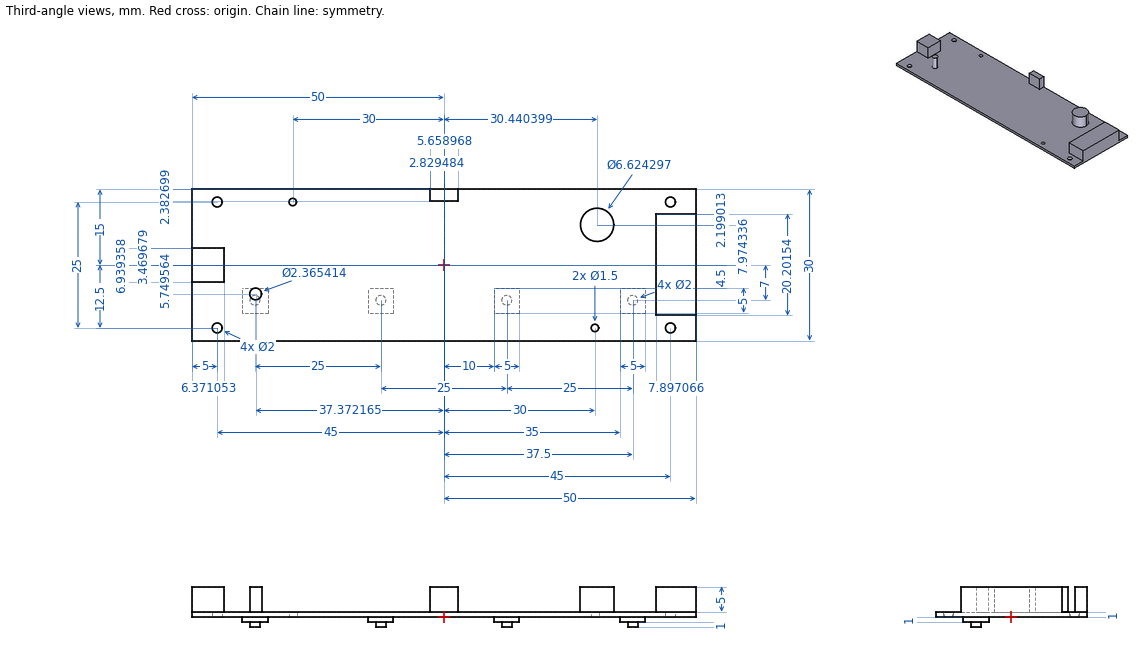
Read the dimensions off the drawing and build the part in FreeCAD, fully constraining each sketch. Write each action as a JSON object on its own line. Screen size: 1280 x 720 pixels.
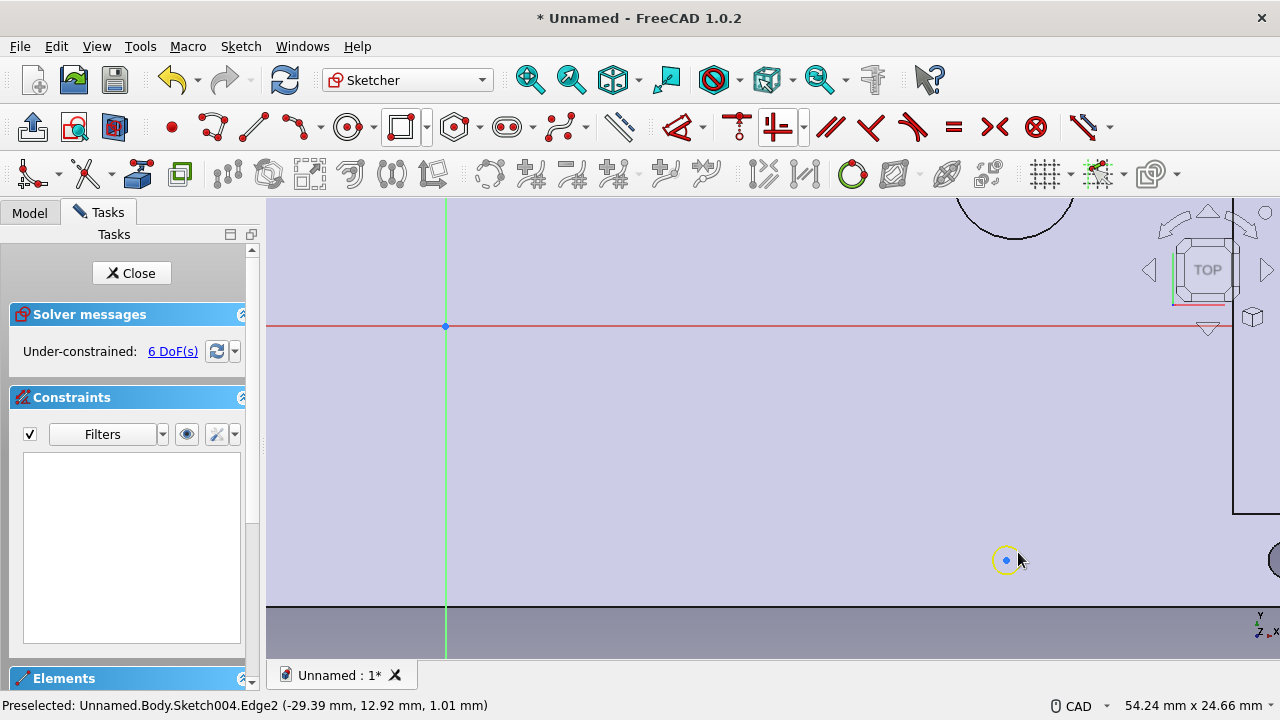
{"action": "left_click", "coordinate": [1017, 550]}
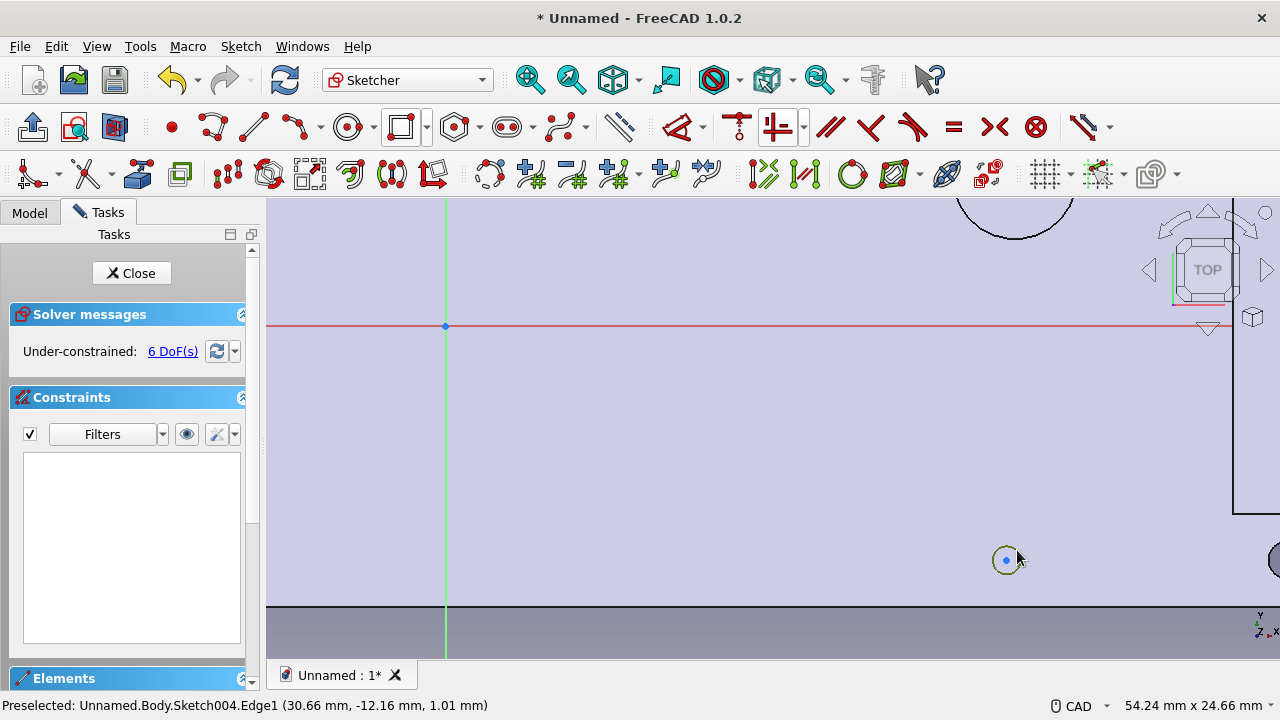
{"action": "scroll", "coordinate": [1019, 553], "scroll_direction": "down", "scroll_amount": 3}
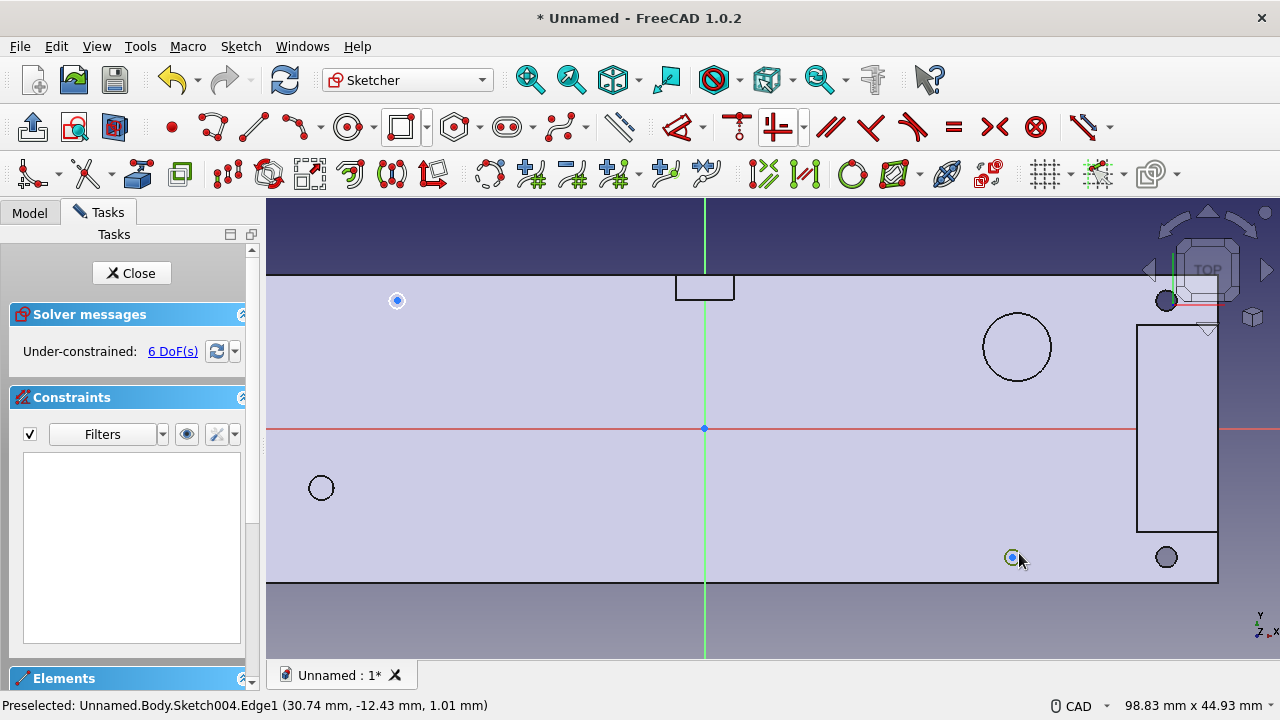
{"action": "scroll", "coordinate": [403, 295], "scroll_direction": "up", "scroll_amount": 3}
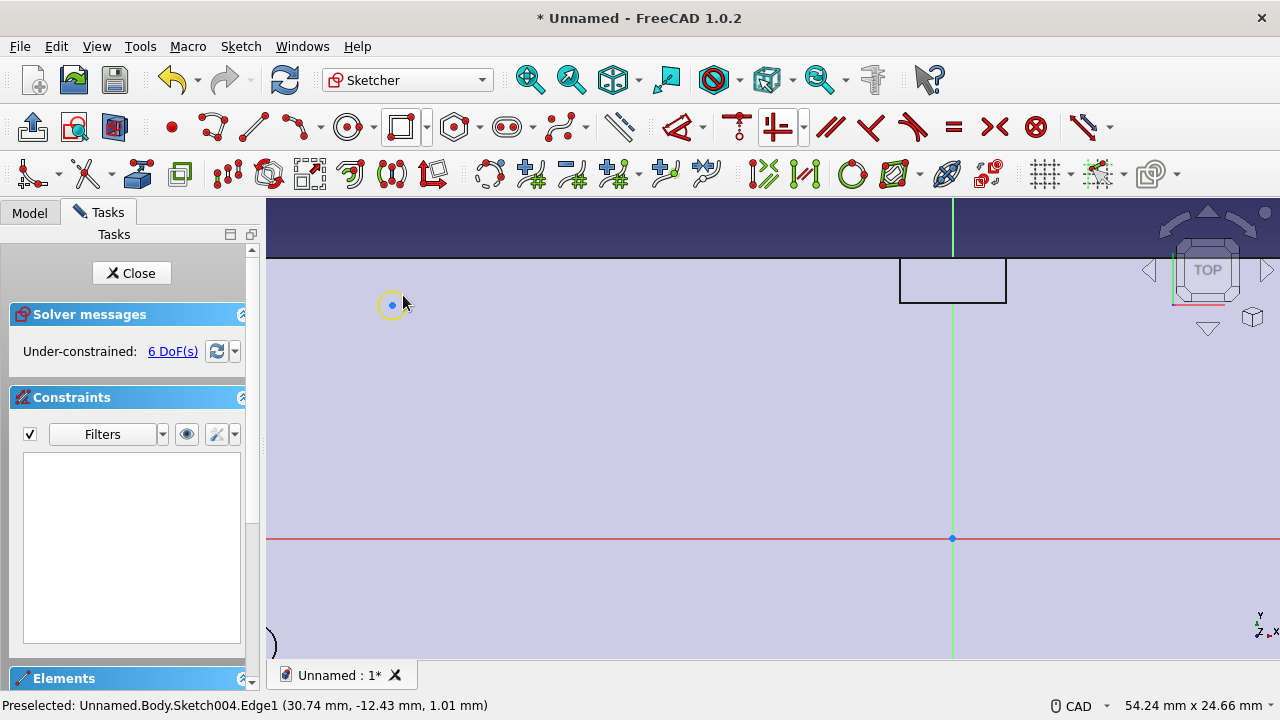
{"action": "left_click", "coordinate": [402, 296]}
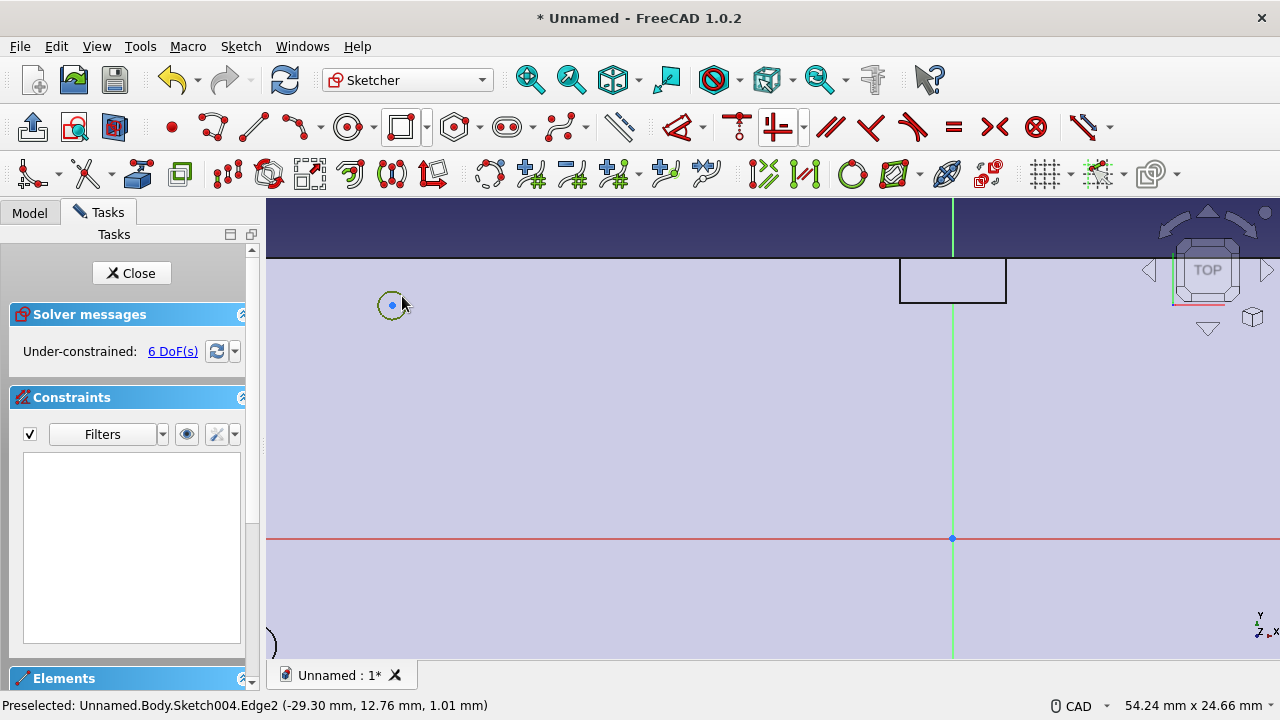
{"action": "left_click", "coordinate": [954, 128]}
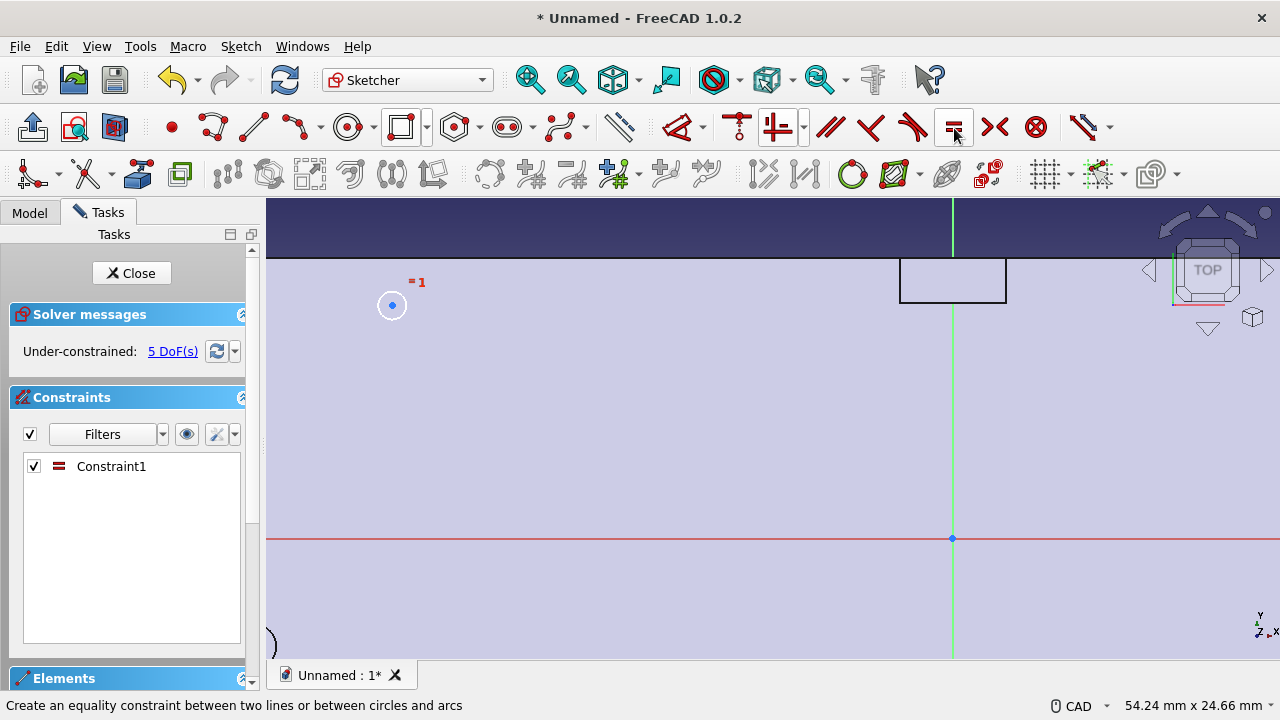
{"action": "key", "text": "d"}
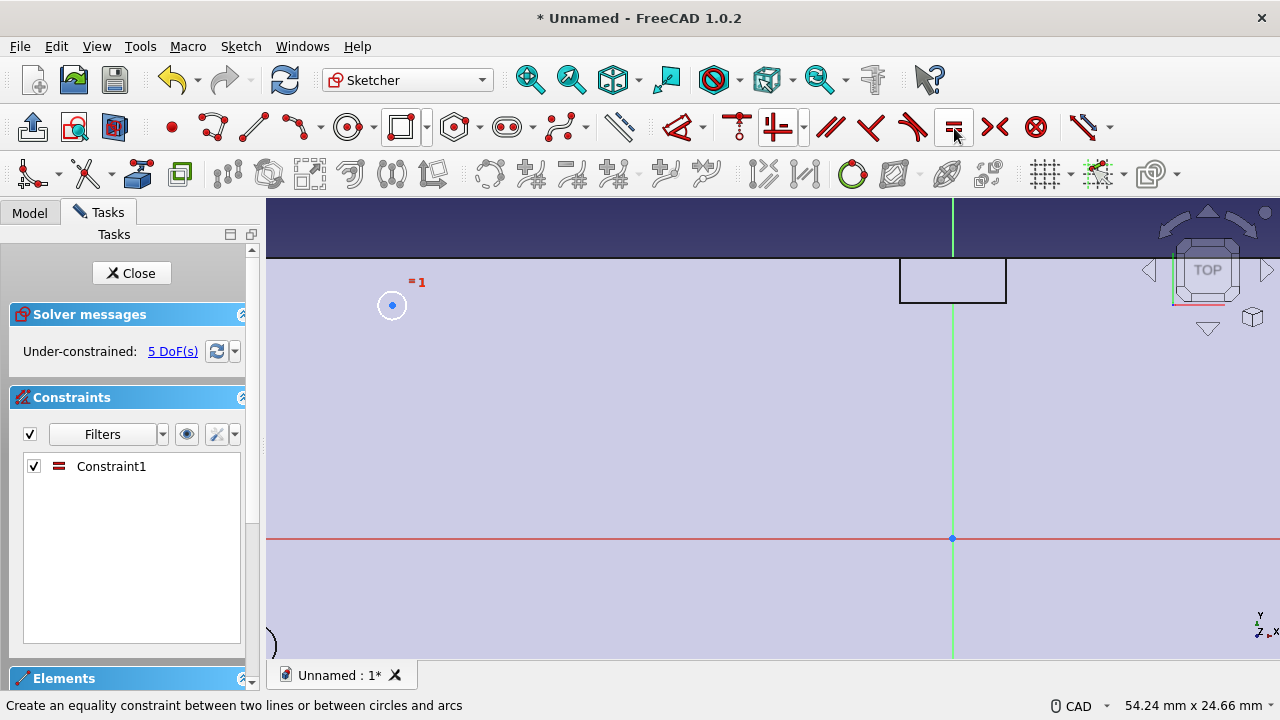
{"action": "scroll", "coordinate": [402, 294], "scroll_direction": "down", "scroll_amount": 3}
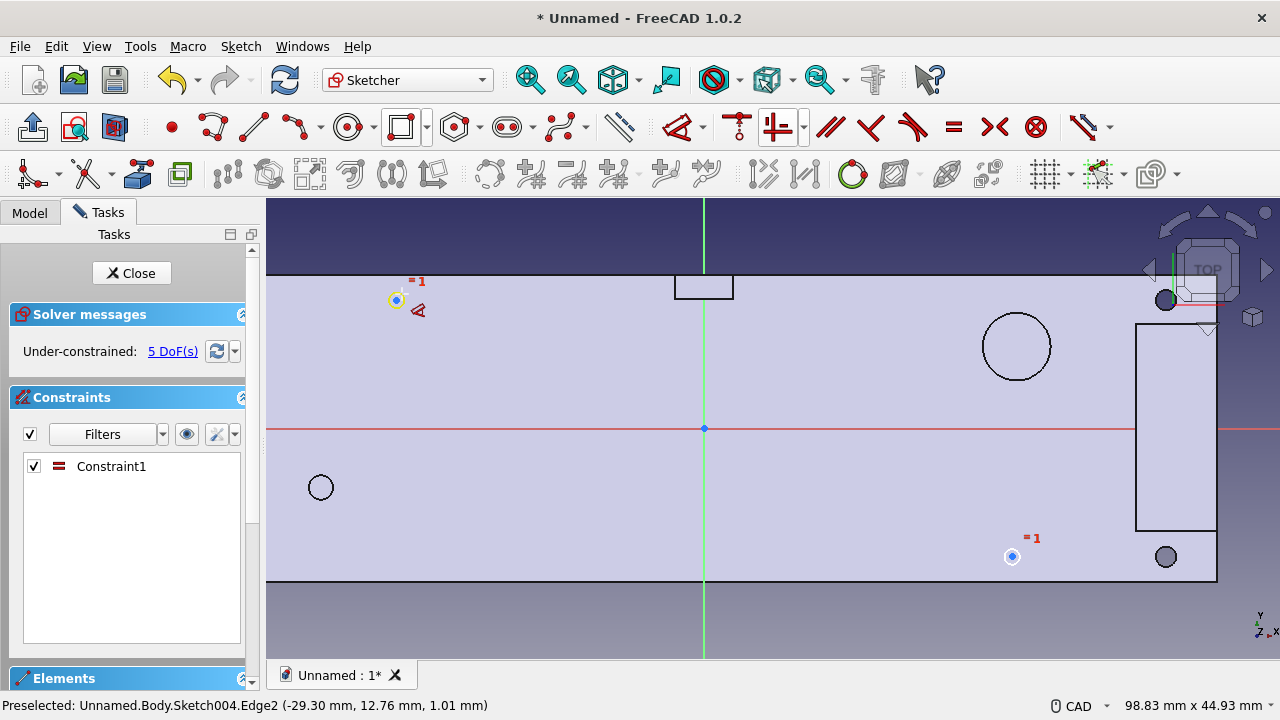
{"action": "scroll", "coordinate": [1018, 552], "scroll_direction": "up", "scroll_amount": 5}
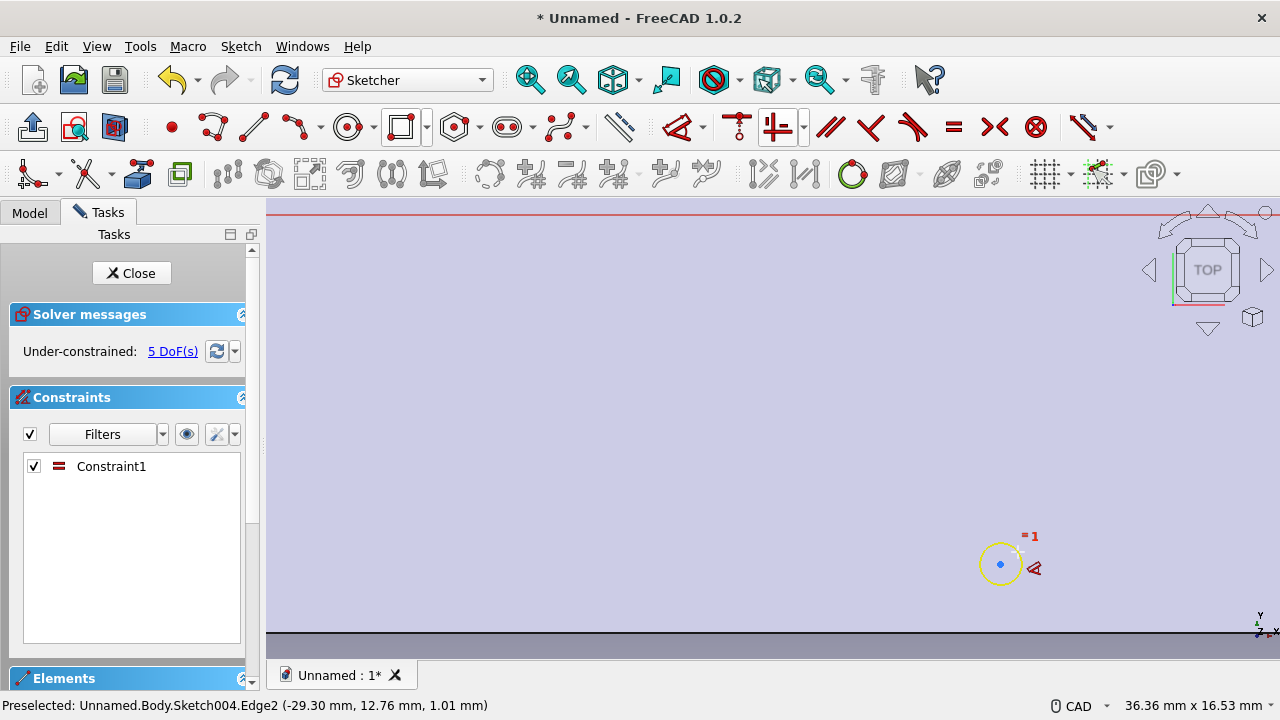
{"action": "left_click", "coordinate": [1016, 549]}
{"action": "left_click", "coordinate": [1039, 526]}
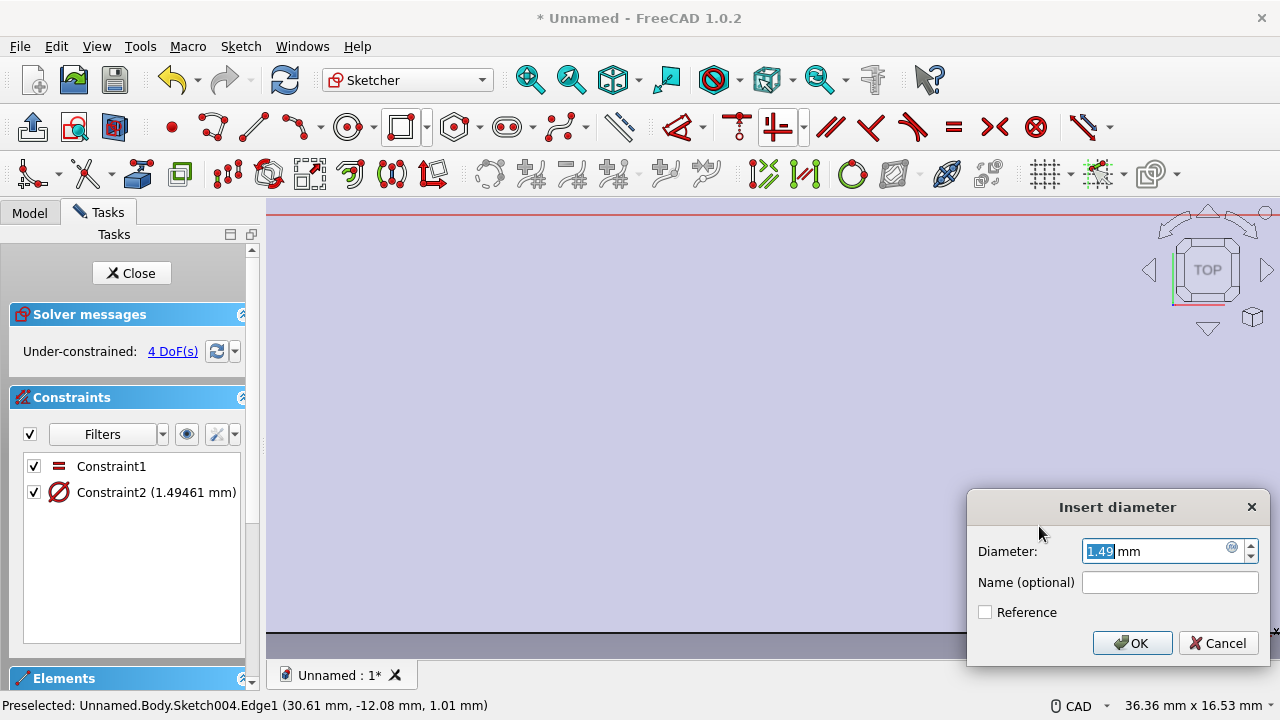
{"action": "type", "text": "1.5"}
{"action": "key", "text": "Return"}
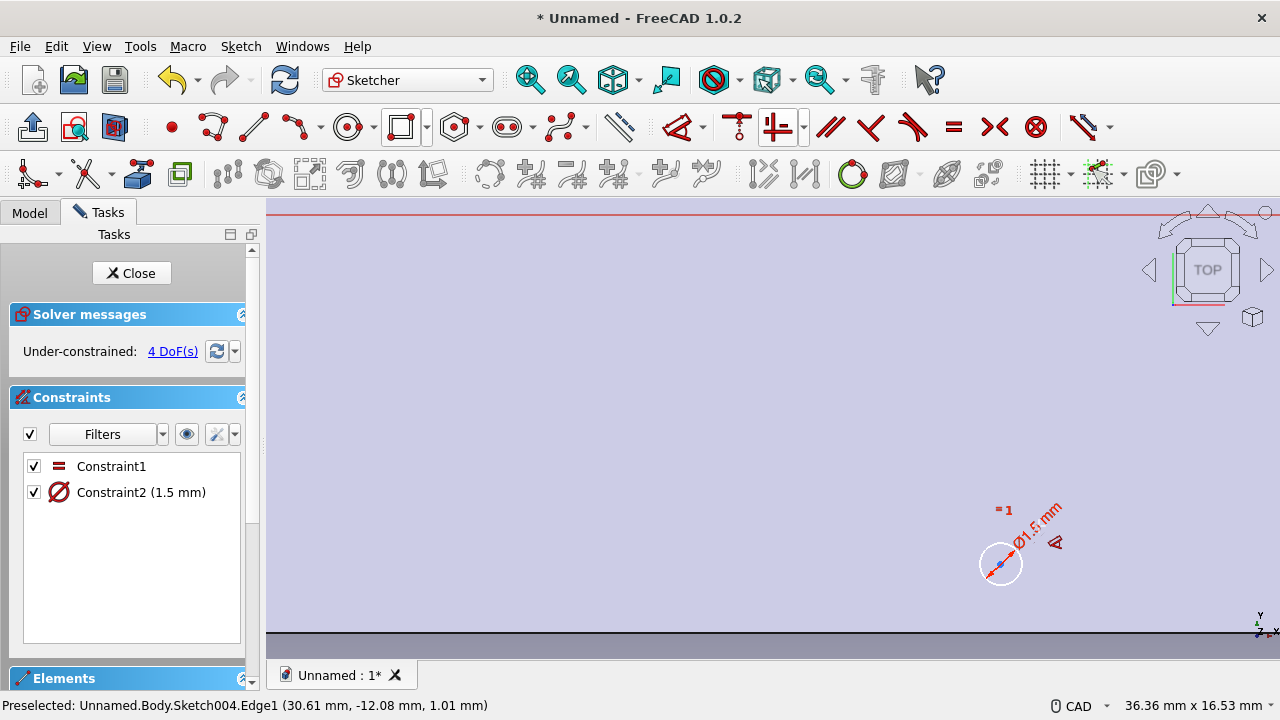
{"action": "left_click", "coordinate": [1001, 564]}
{"action": "left_click", "coordinate": [647, 598]}